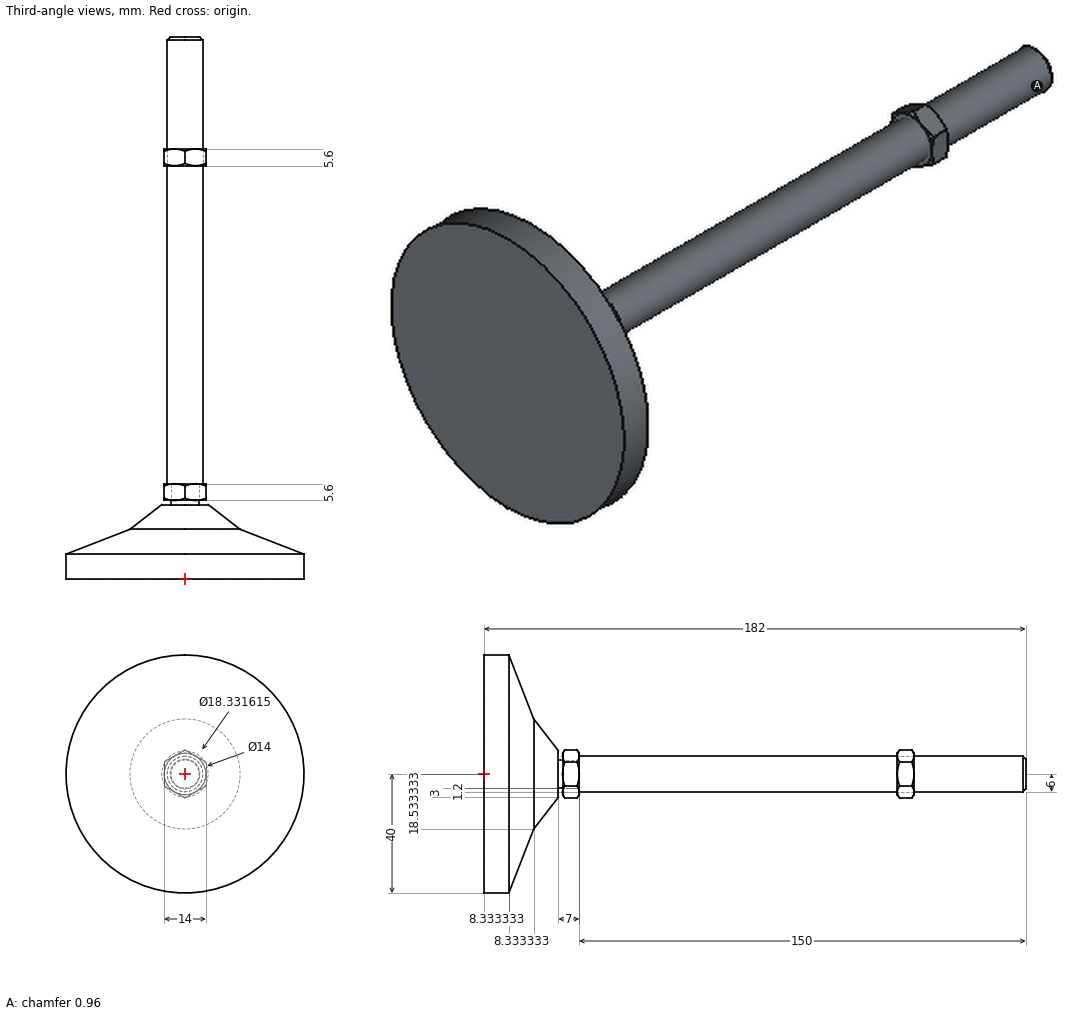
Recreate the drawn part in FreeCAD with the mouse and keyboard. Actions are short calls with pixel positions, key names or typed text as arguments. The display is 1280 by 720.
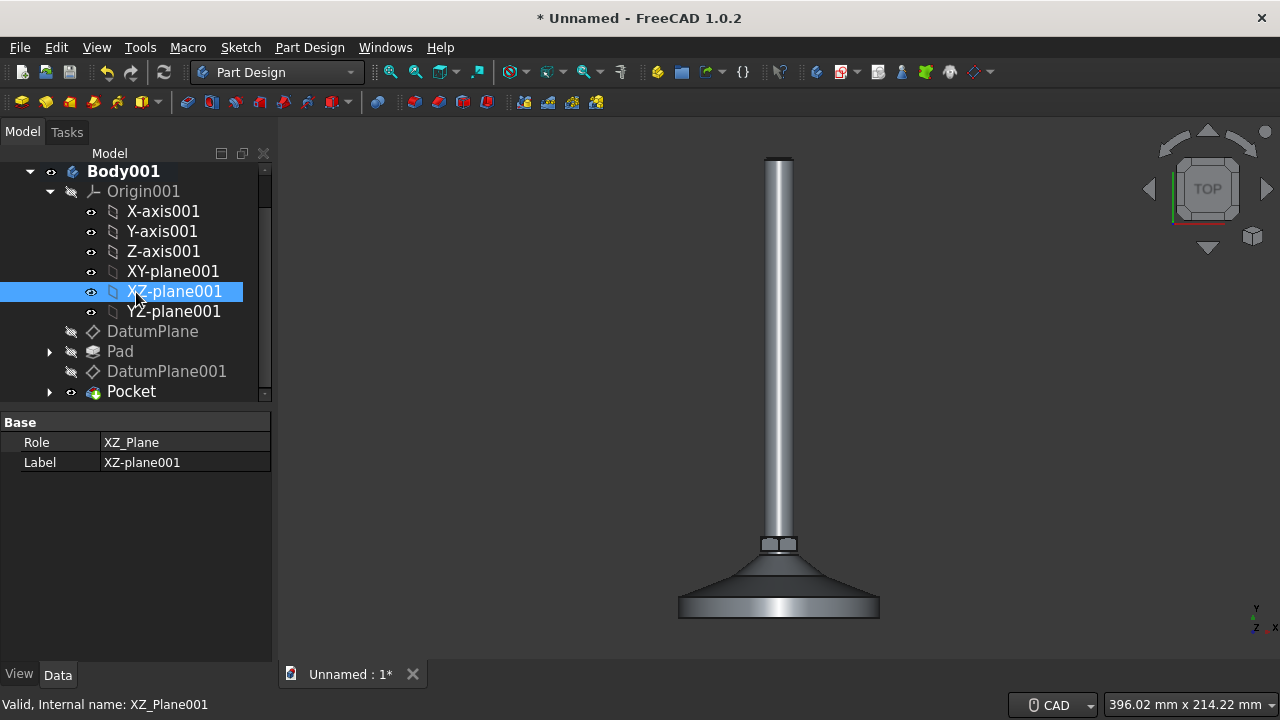
click(974, 72)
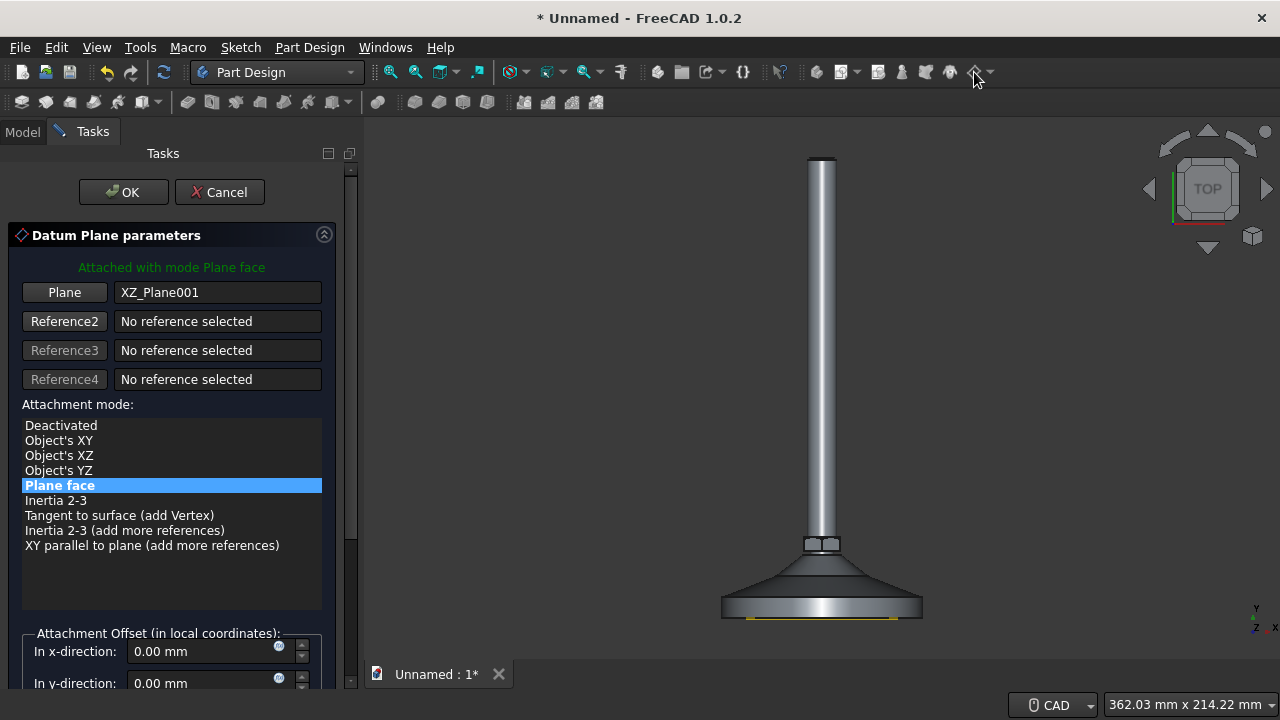
scroll(351, 426, down, 2)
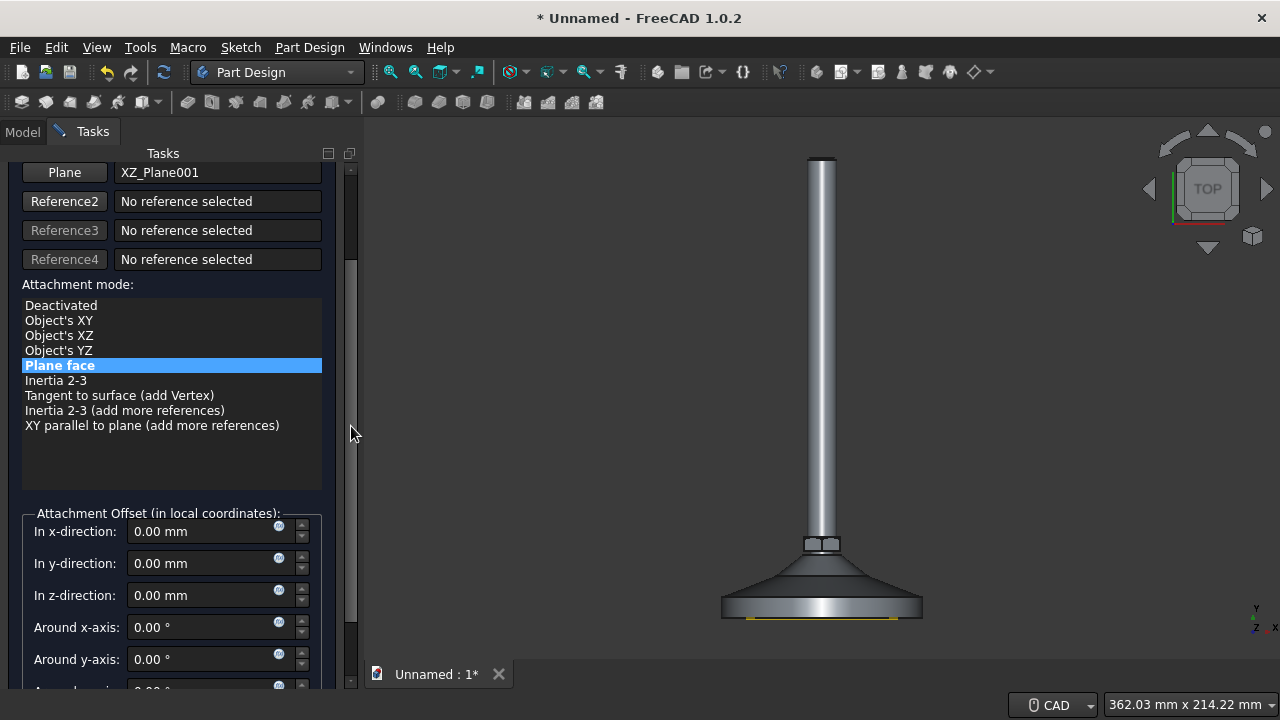
triple_click(210, 595)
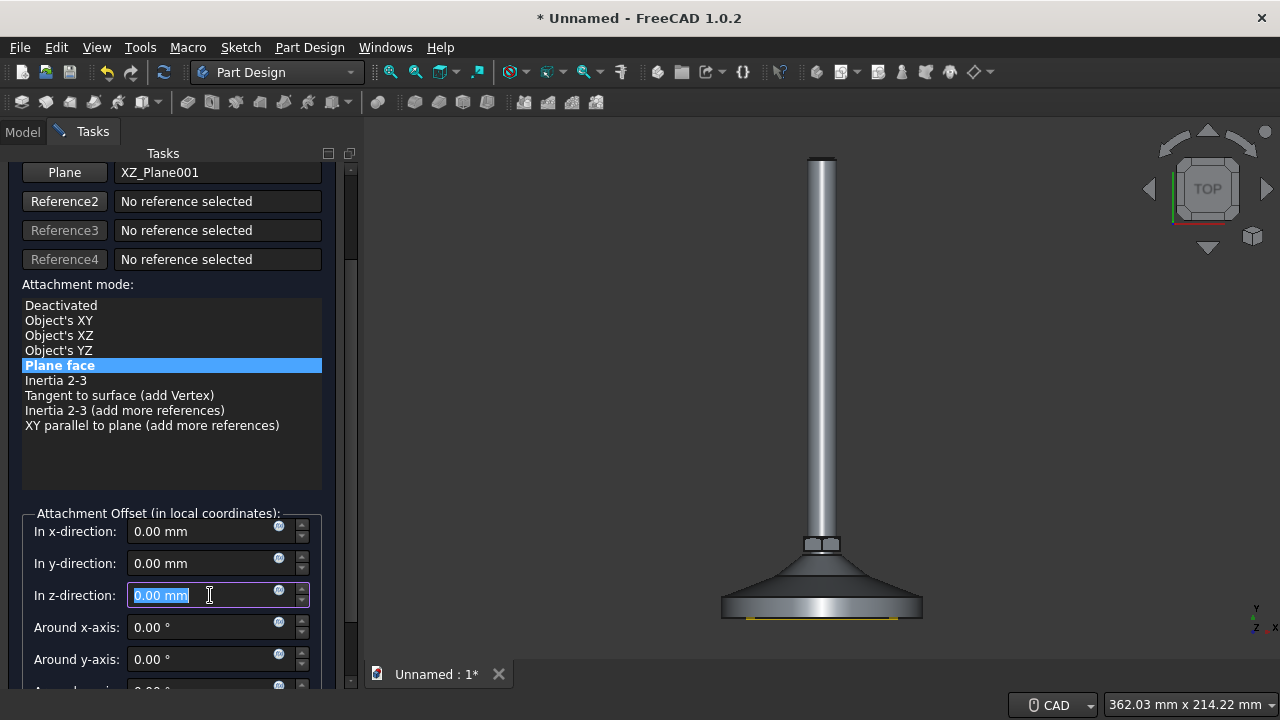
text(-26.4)
key(Tab)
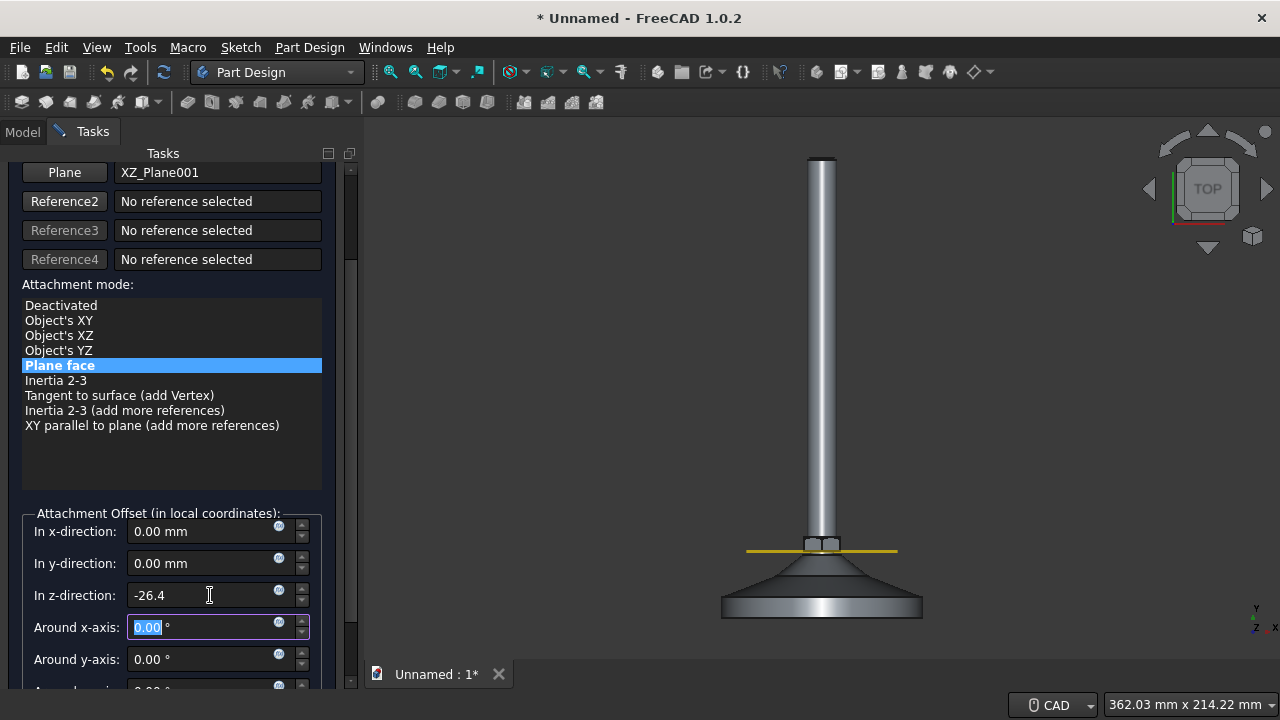
scroll(351, 426, up, 3)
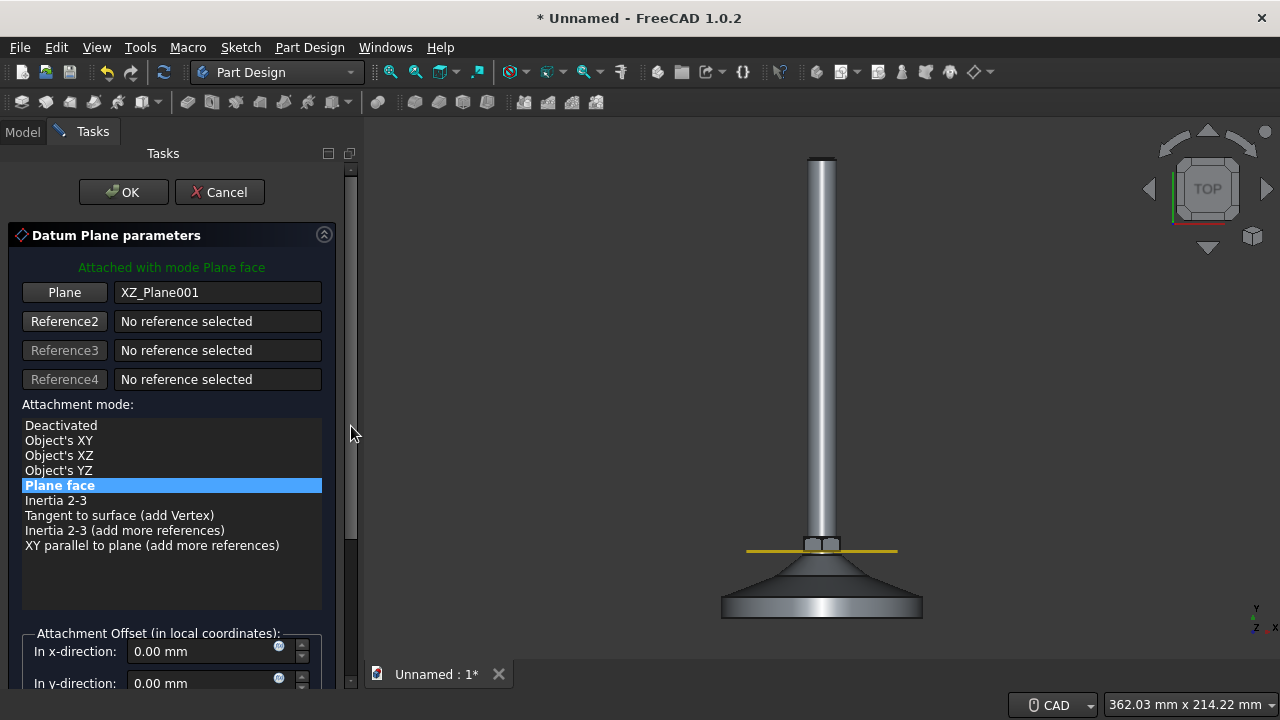
click(124, 192)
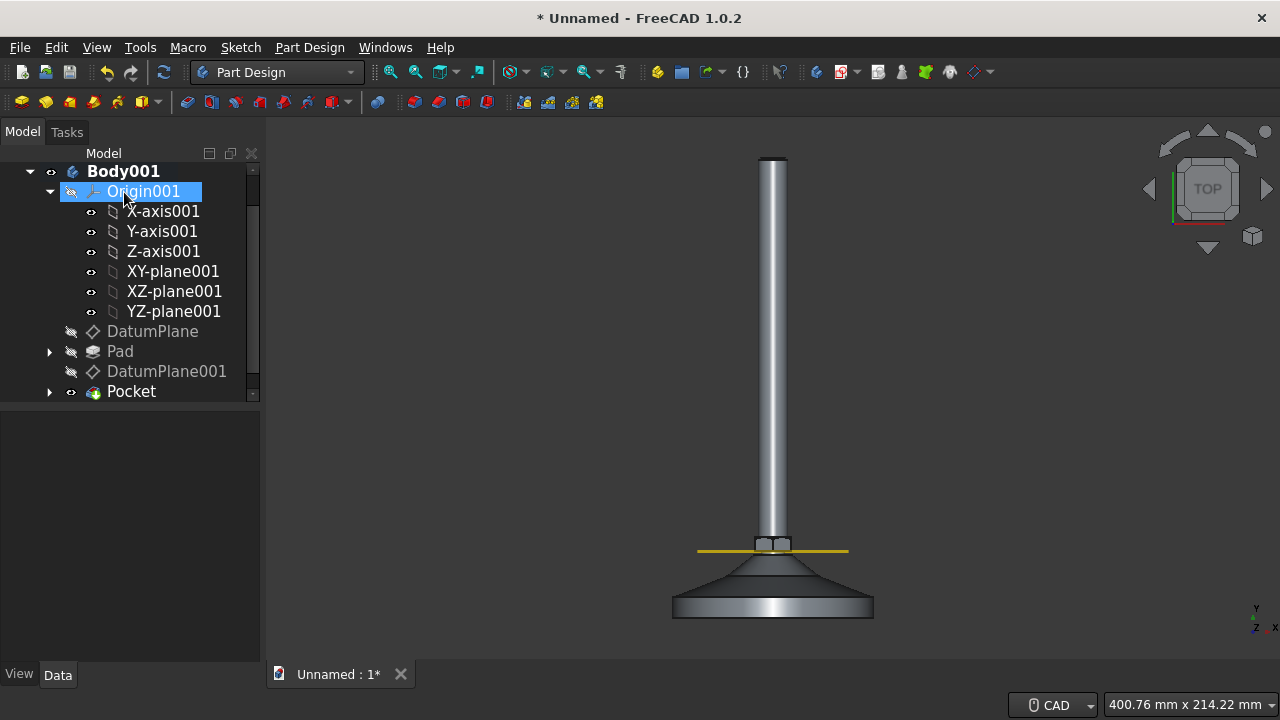
scroll(120, 287, down, 3)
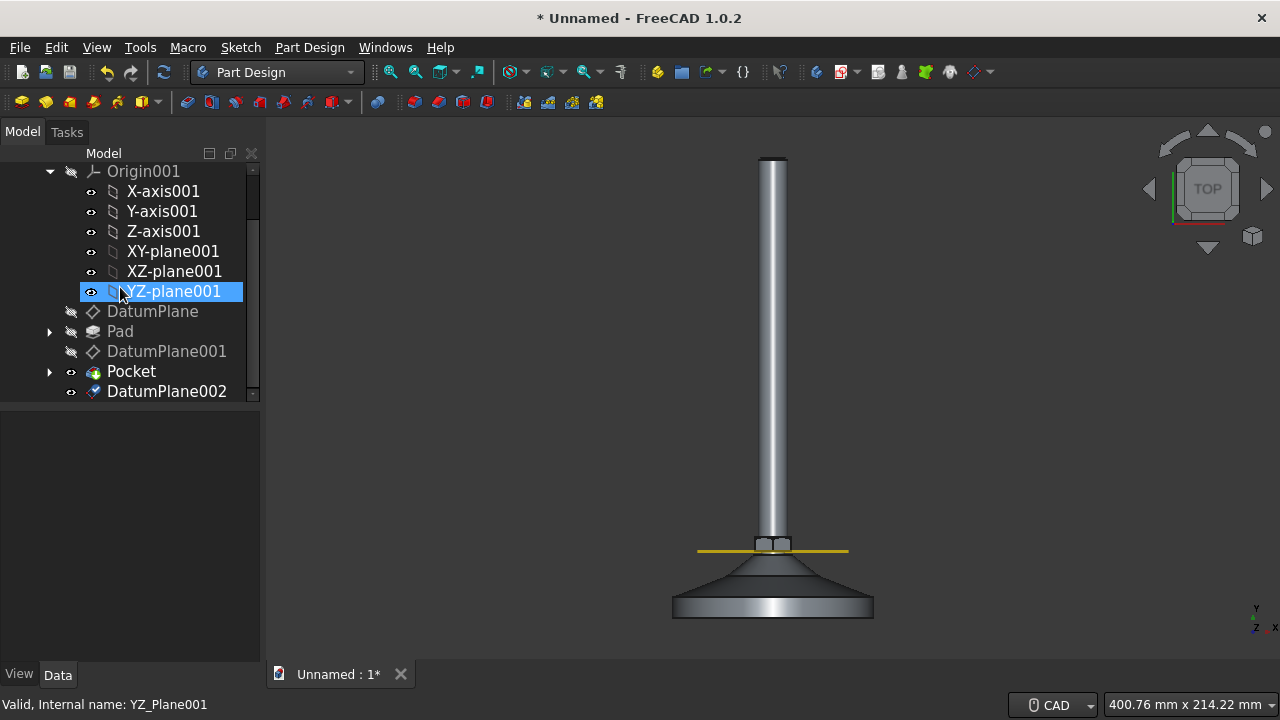
click(116, 392)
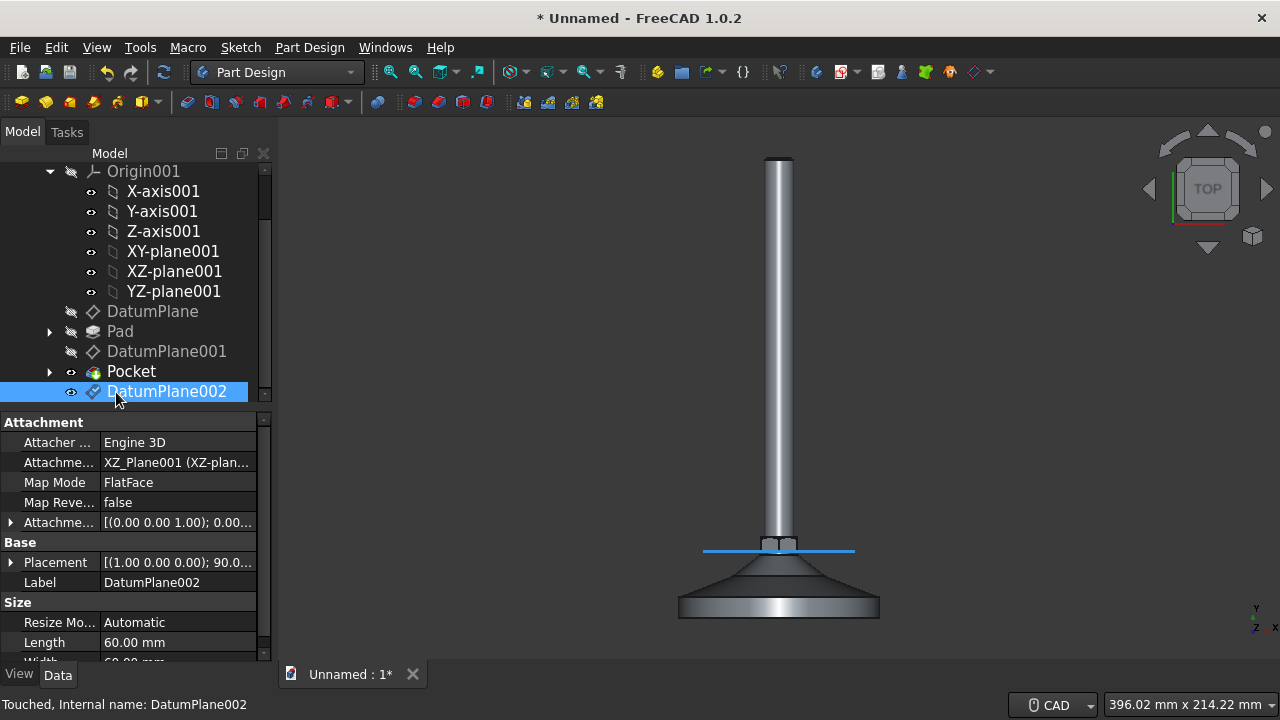
click(842, 72)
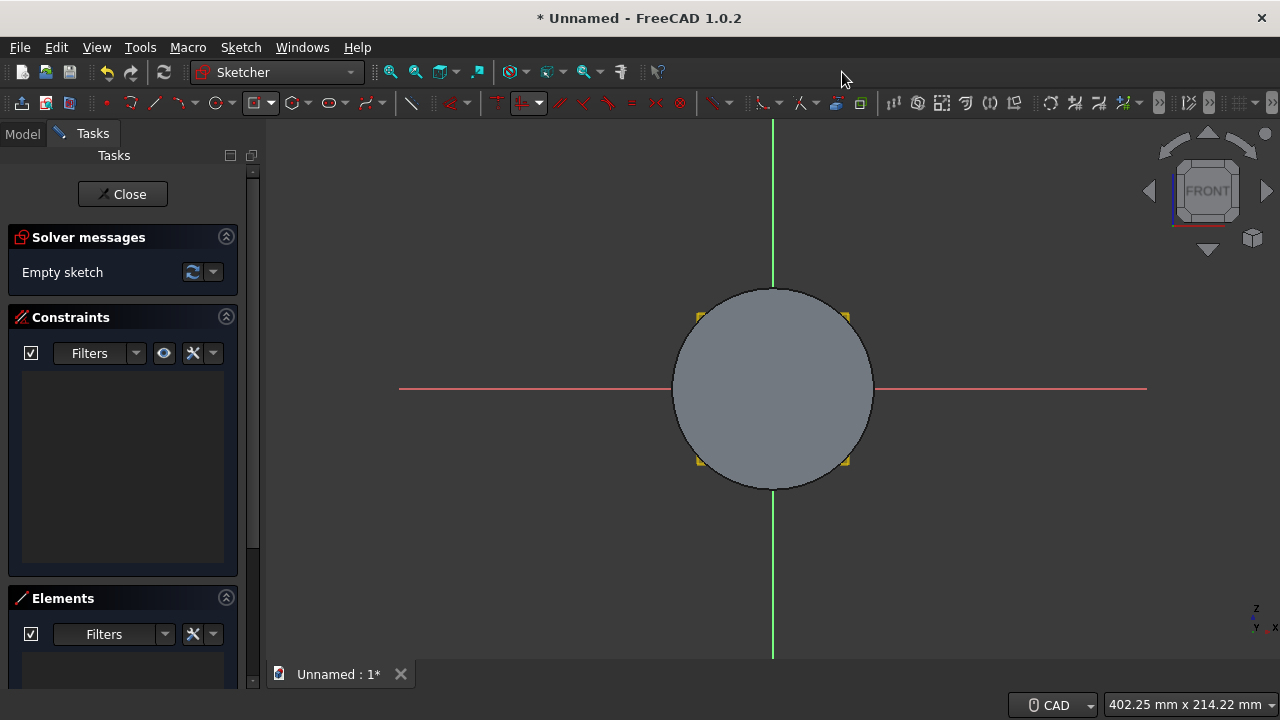
scroll(784, 389, up, 10)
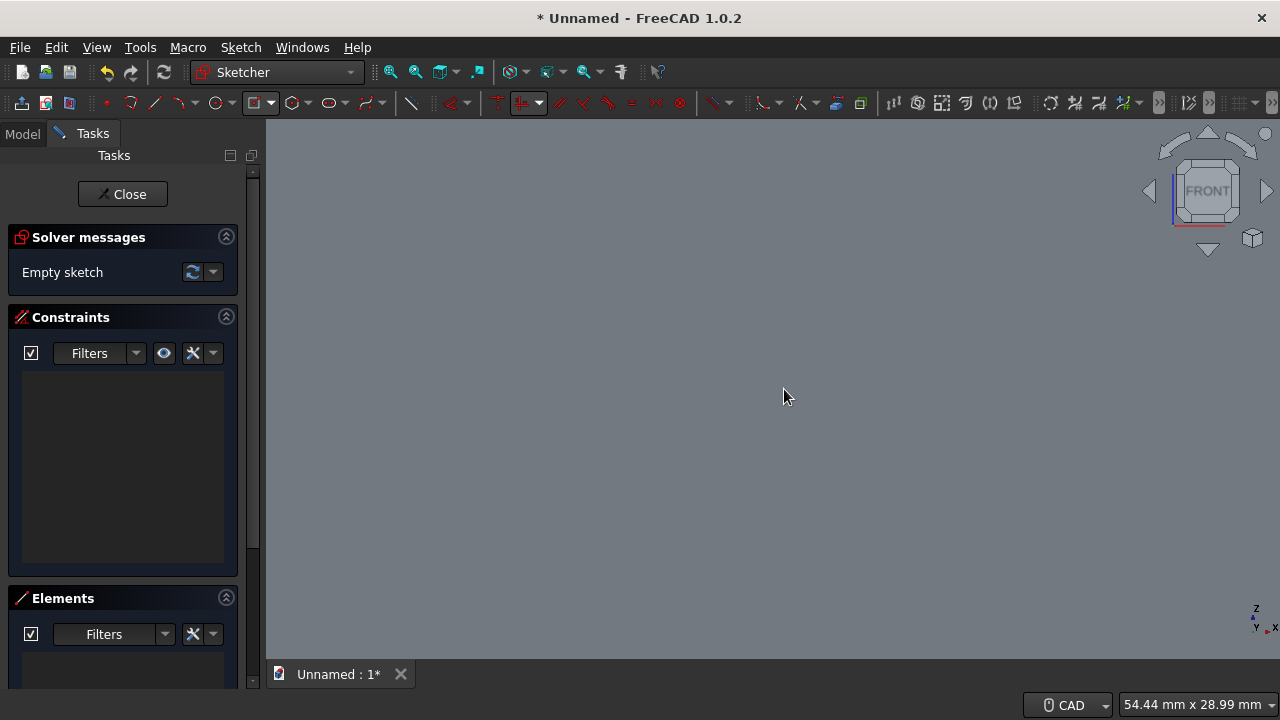
click(216, 104)